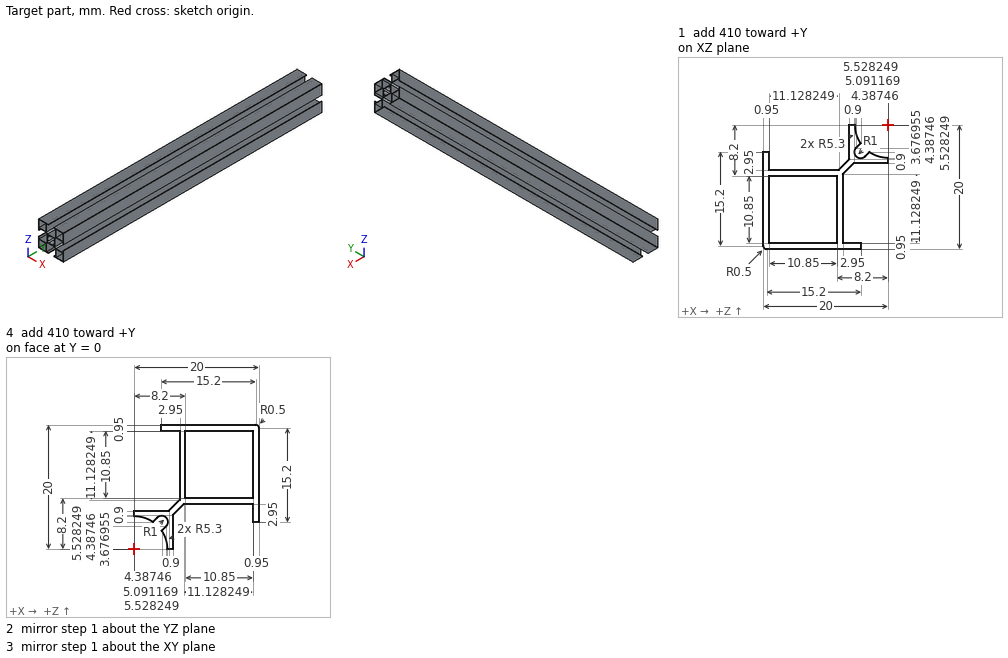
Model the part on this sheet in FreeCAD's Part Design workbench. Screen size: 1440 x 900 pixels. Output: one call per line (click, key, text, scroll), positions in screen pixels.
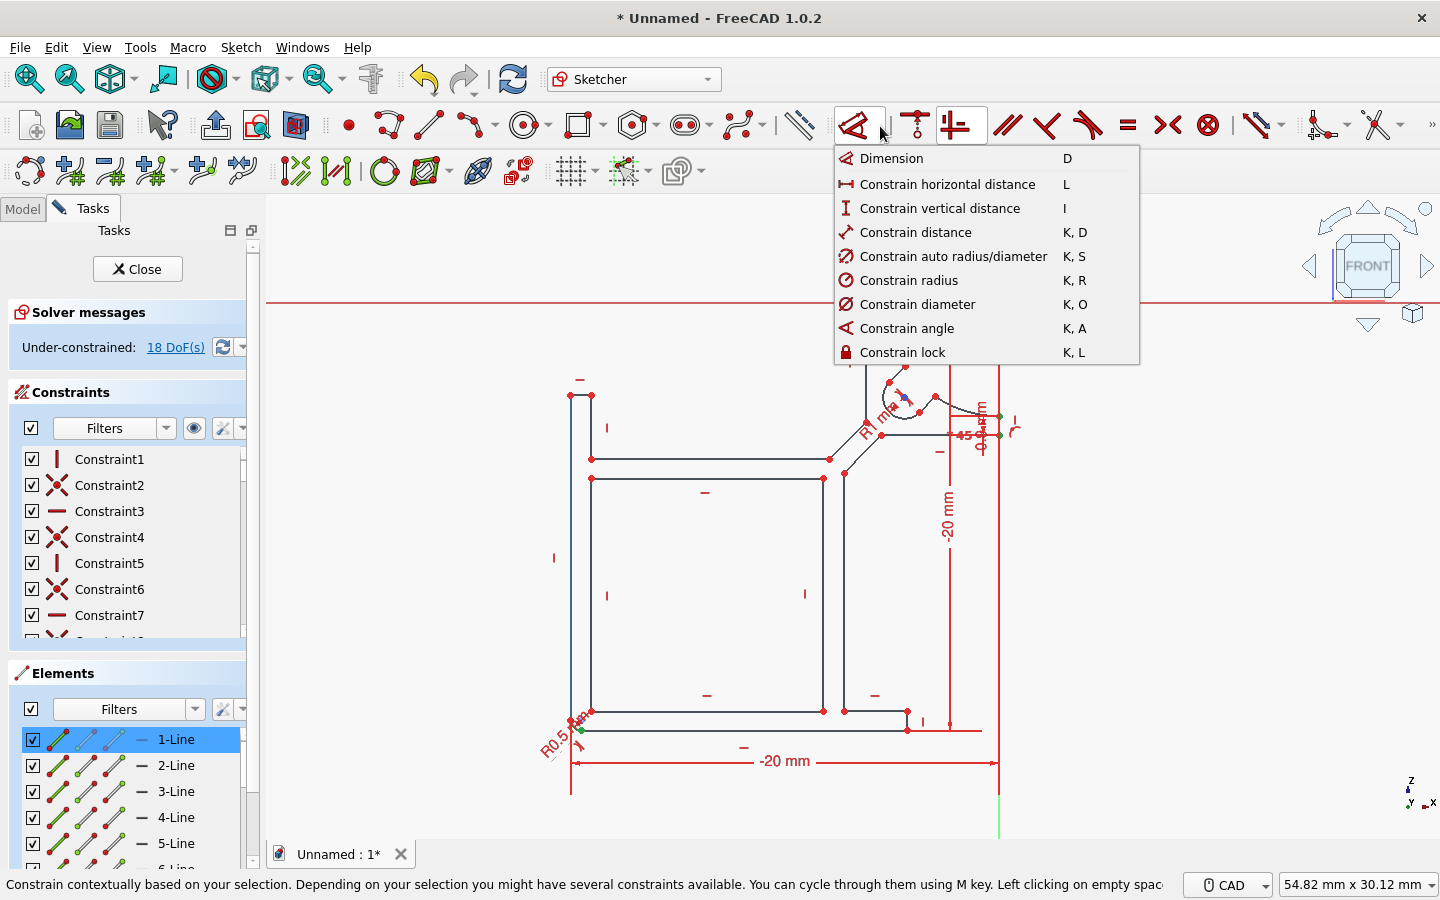
click(987, 208)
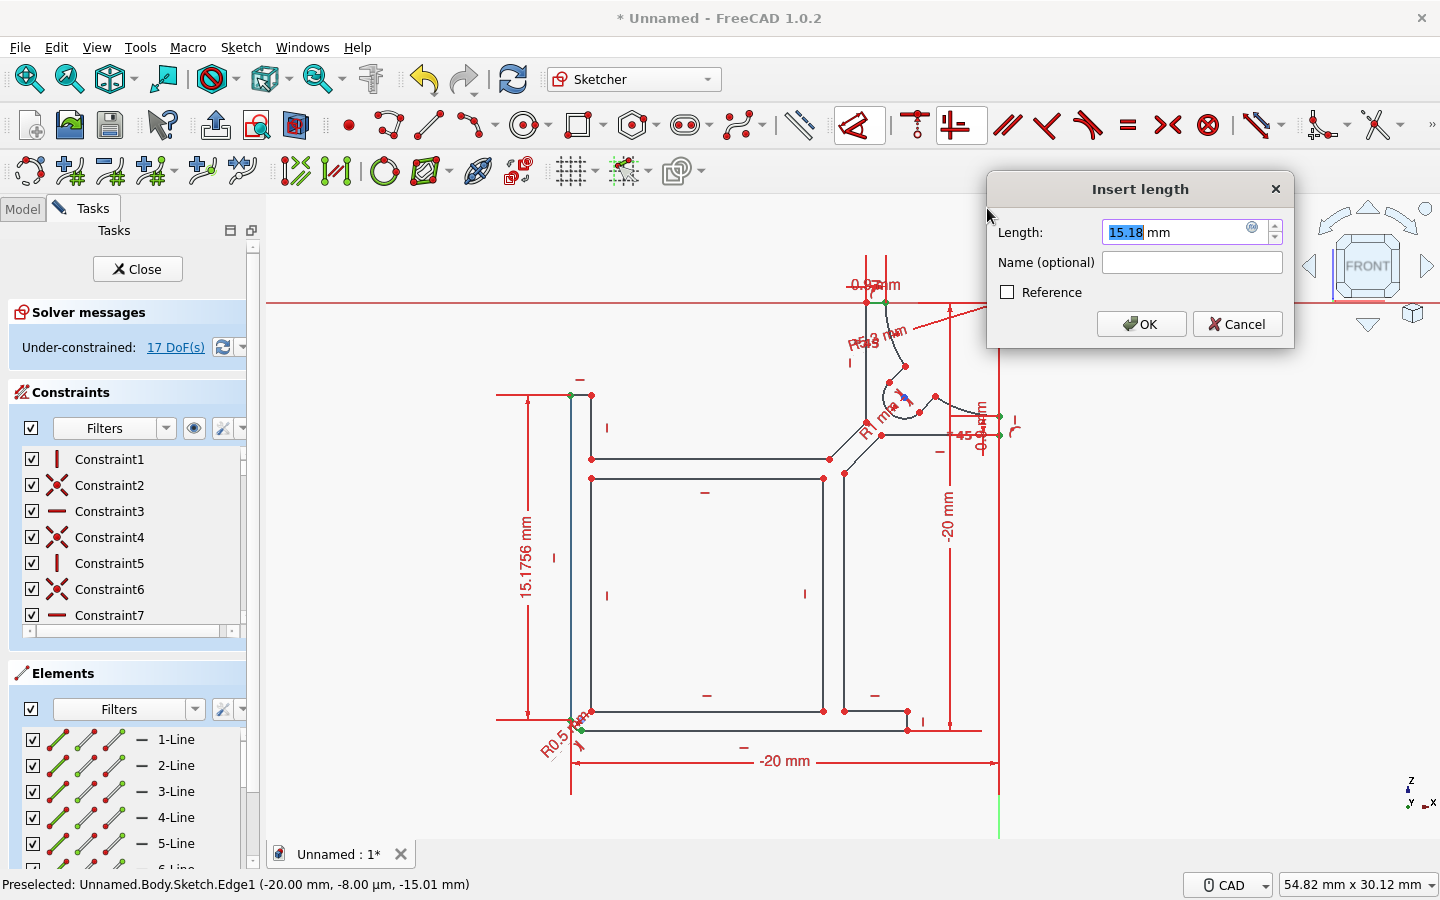
text(15.2)
key(Return)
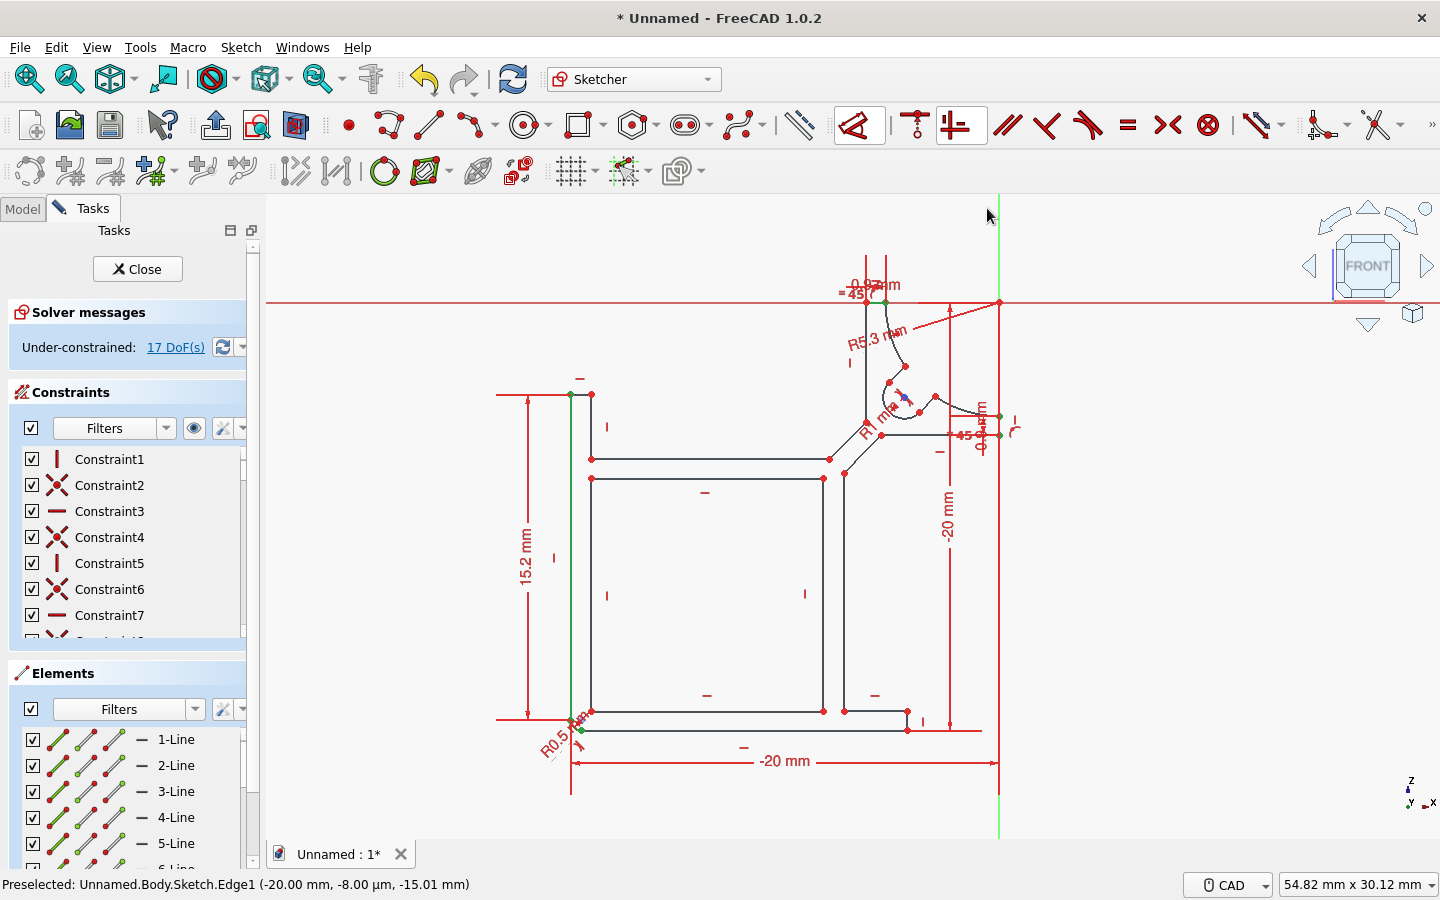
scroll(581, 395, up, 4)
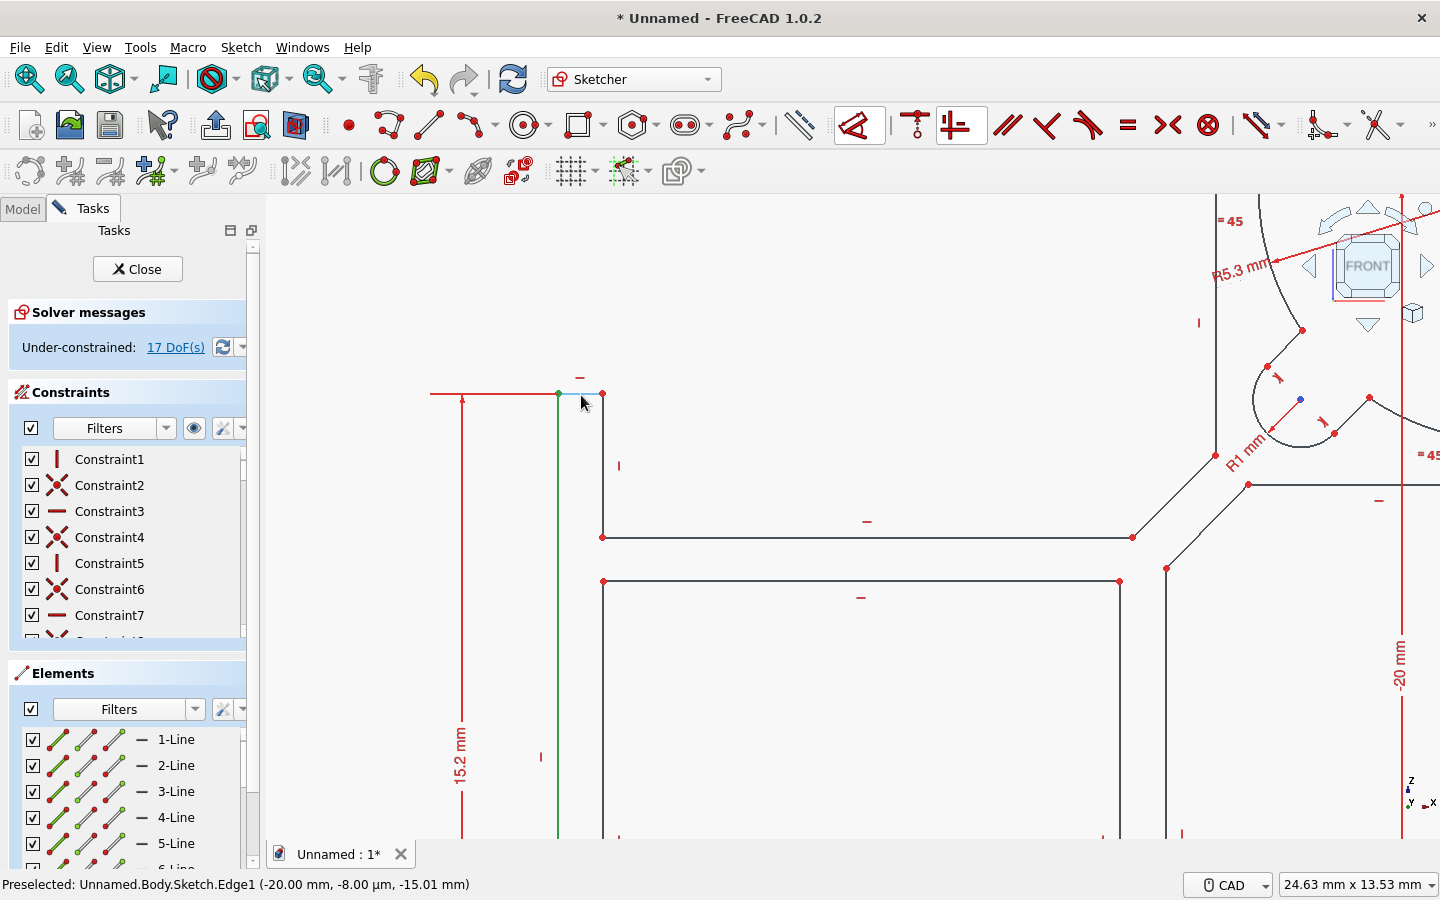
click(581, 394)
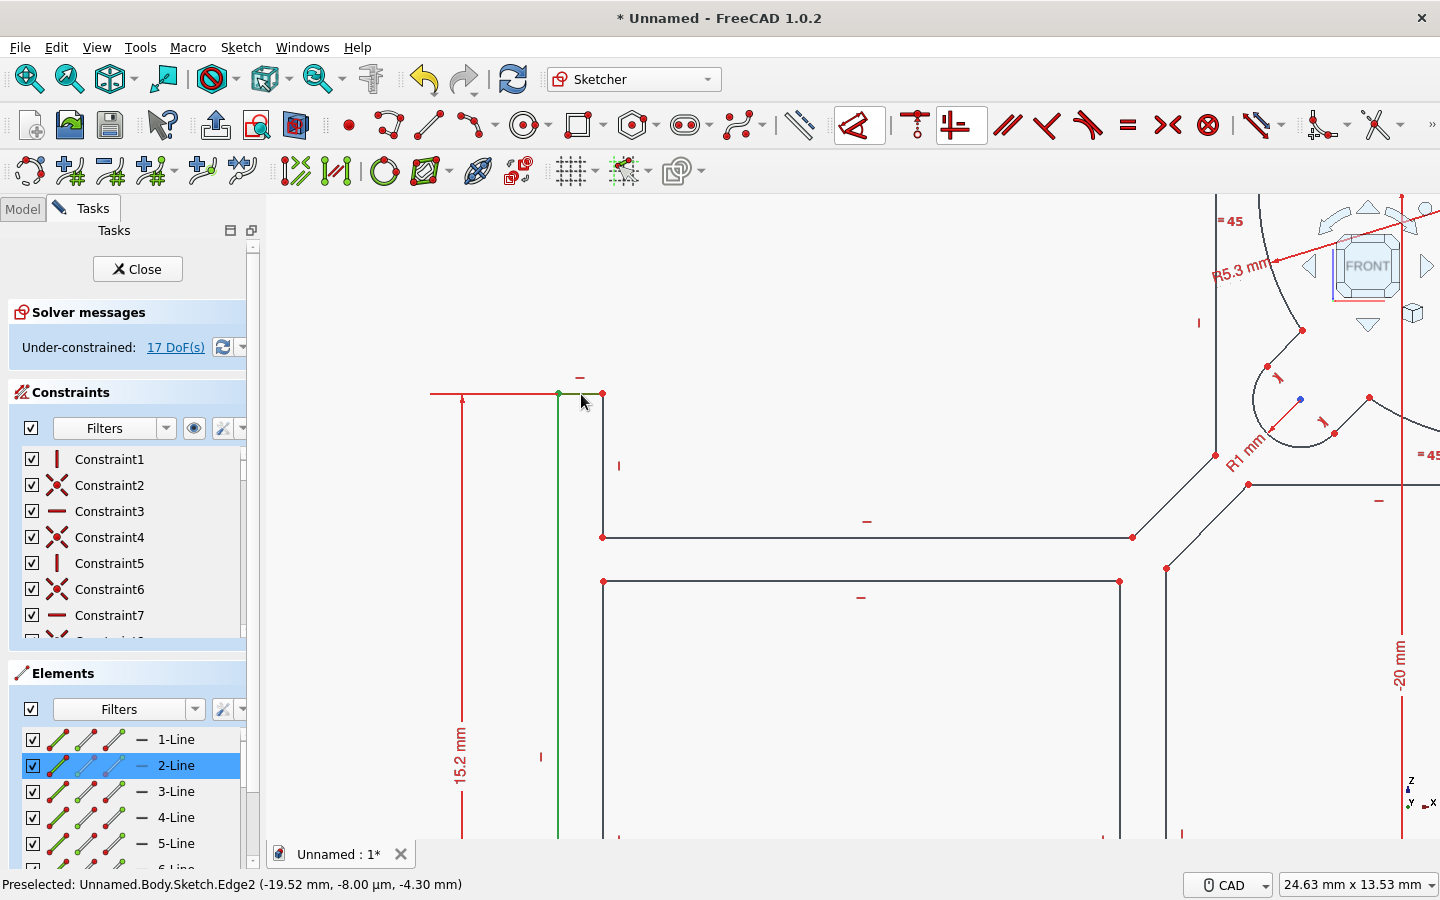
click(880, 126)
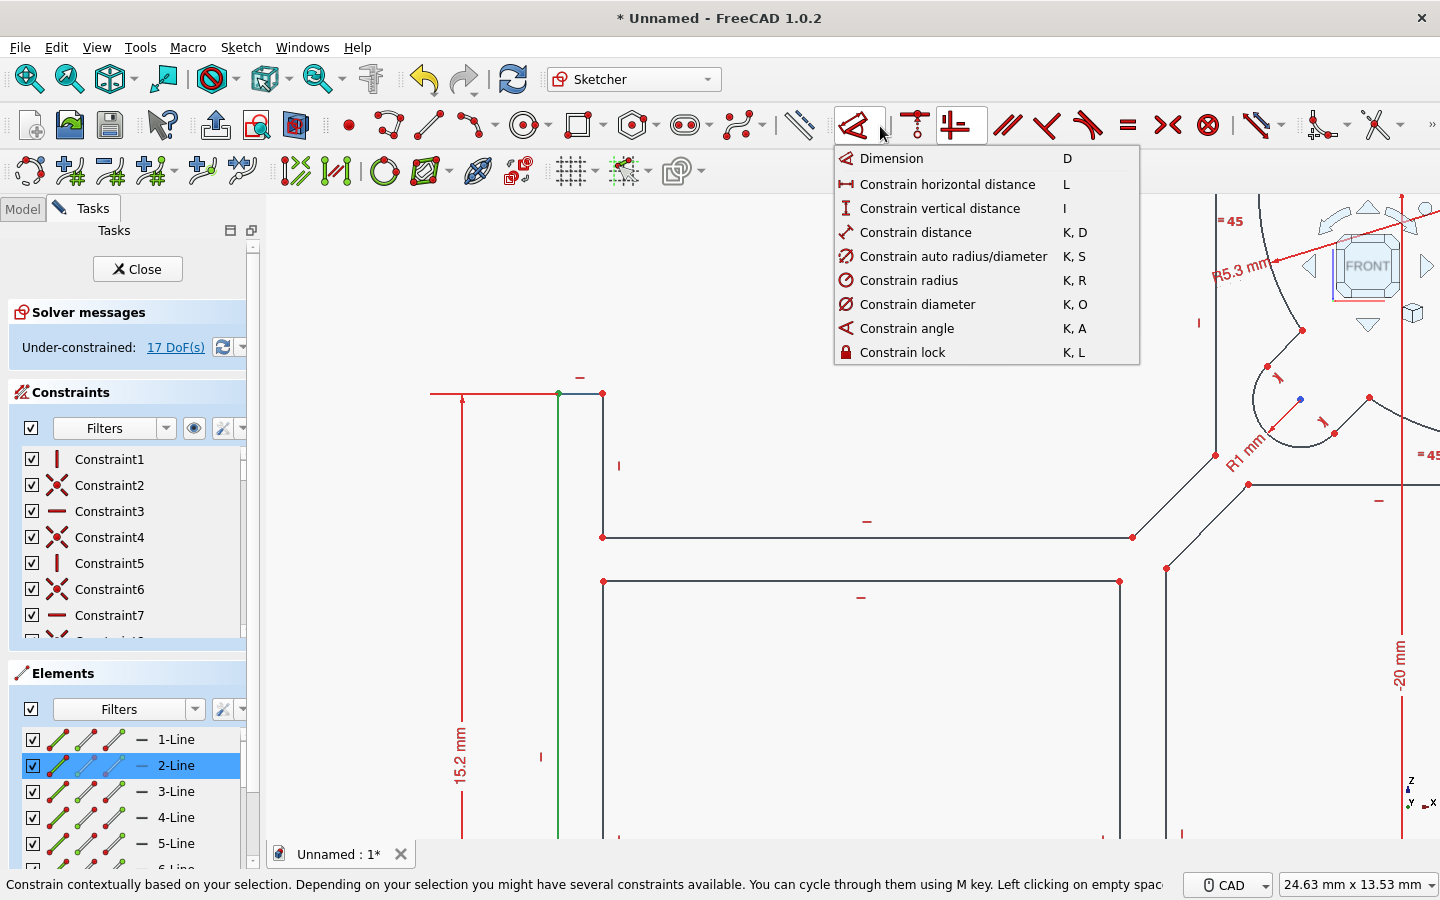
click(987, 184)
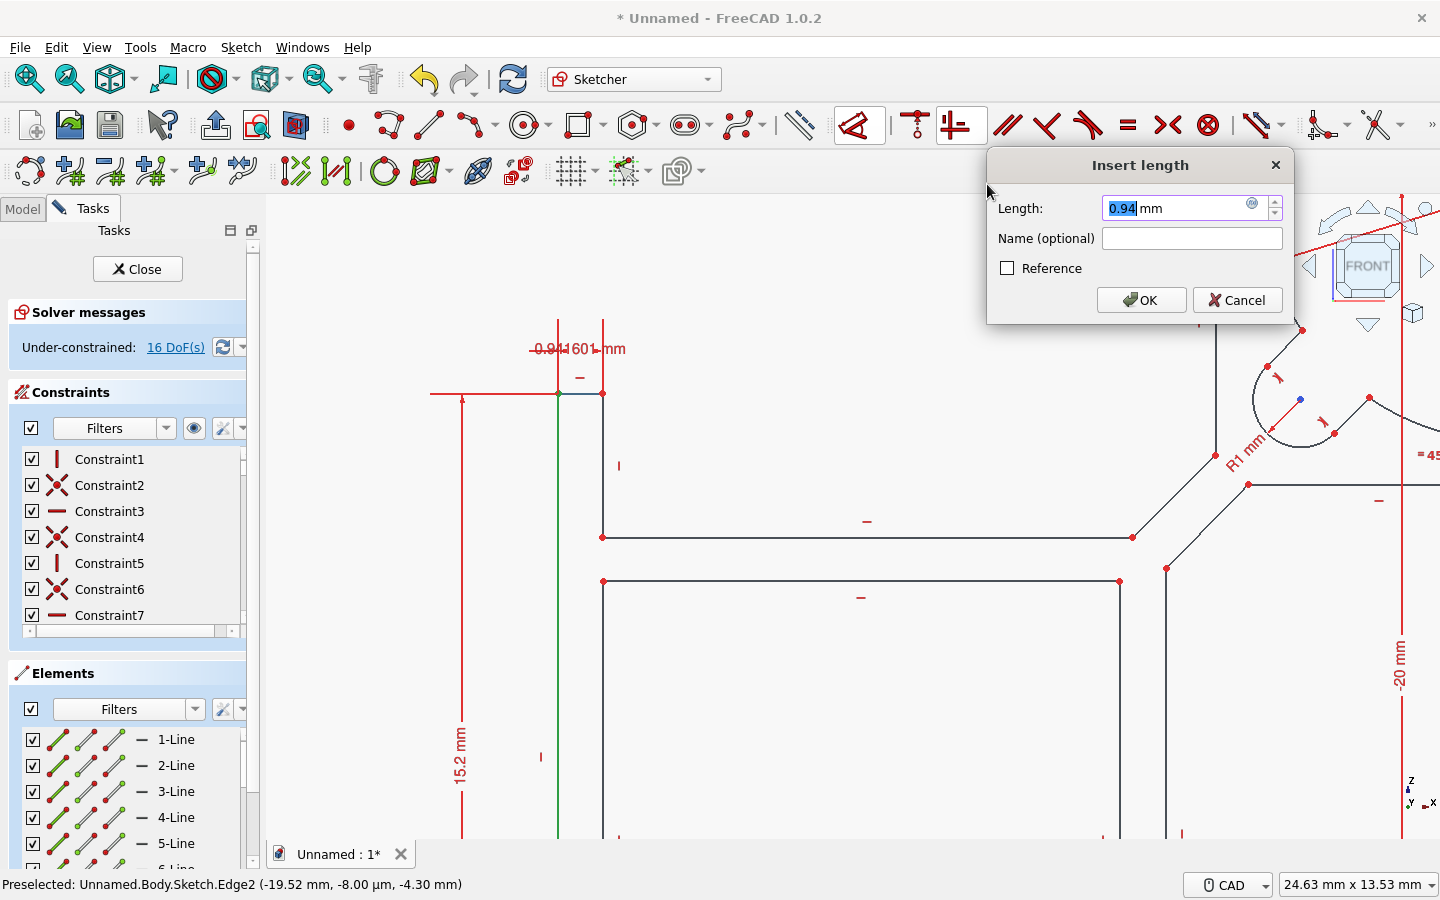
text(0.95)
key(Return)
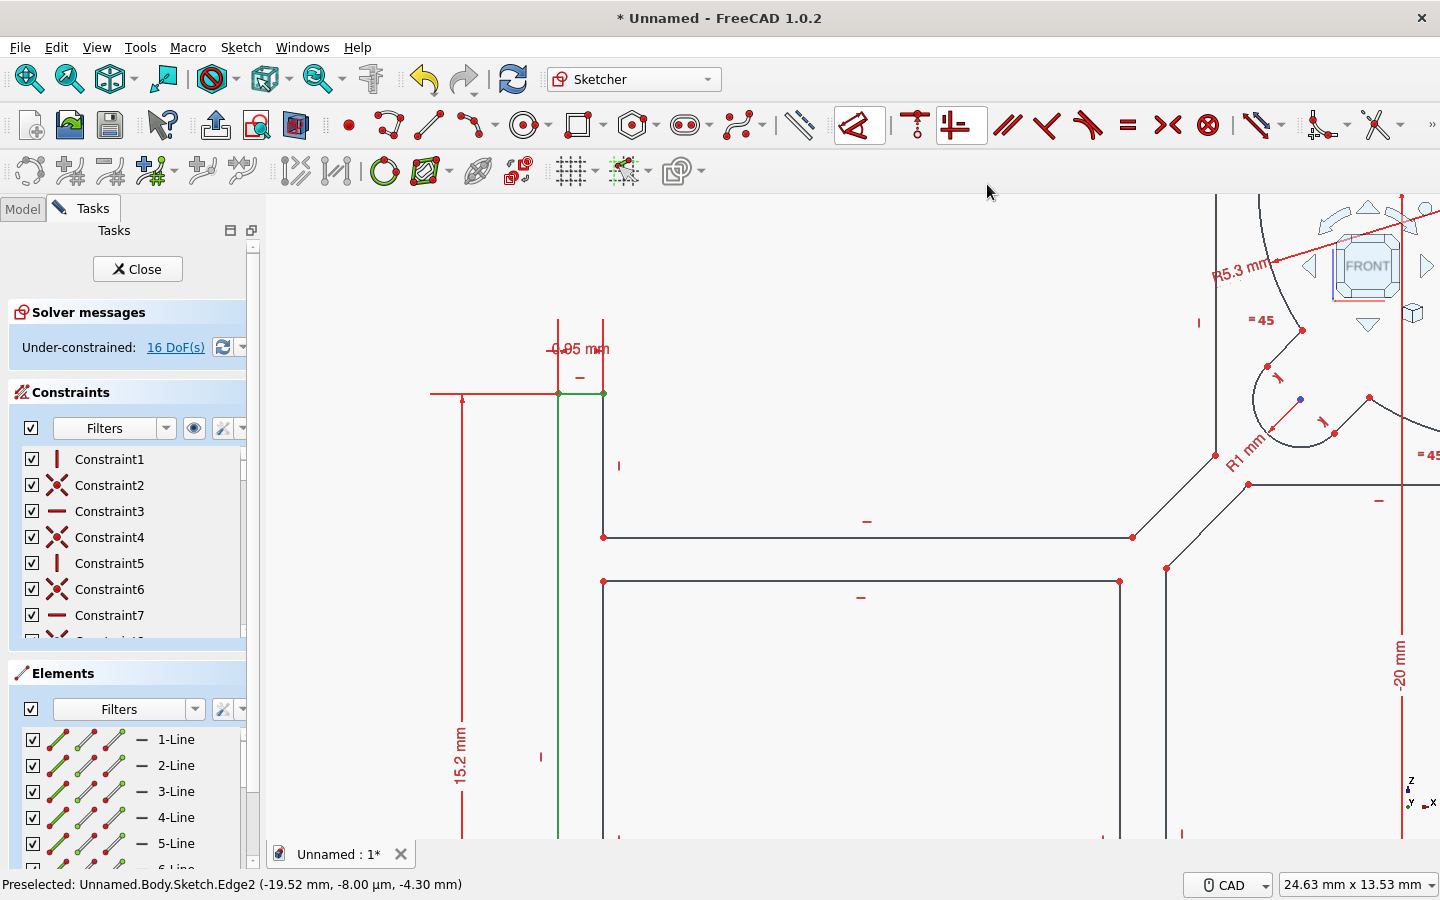
click(603, 437)